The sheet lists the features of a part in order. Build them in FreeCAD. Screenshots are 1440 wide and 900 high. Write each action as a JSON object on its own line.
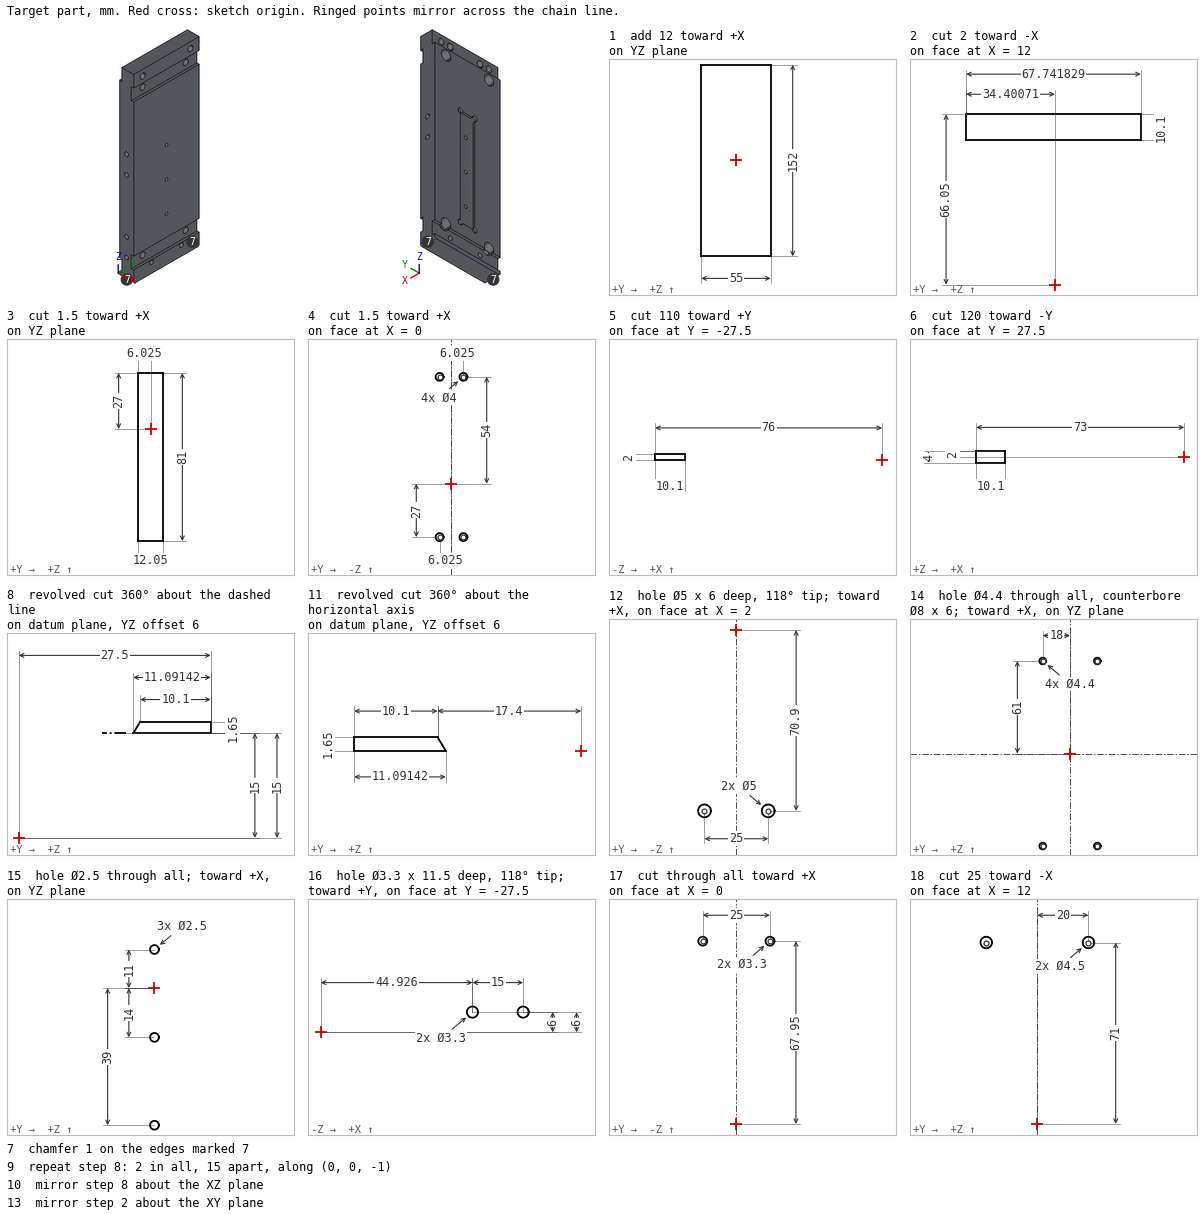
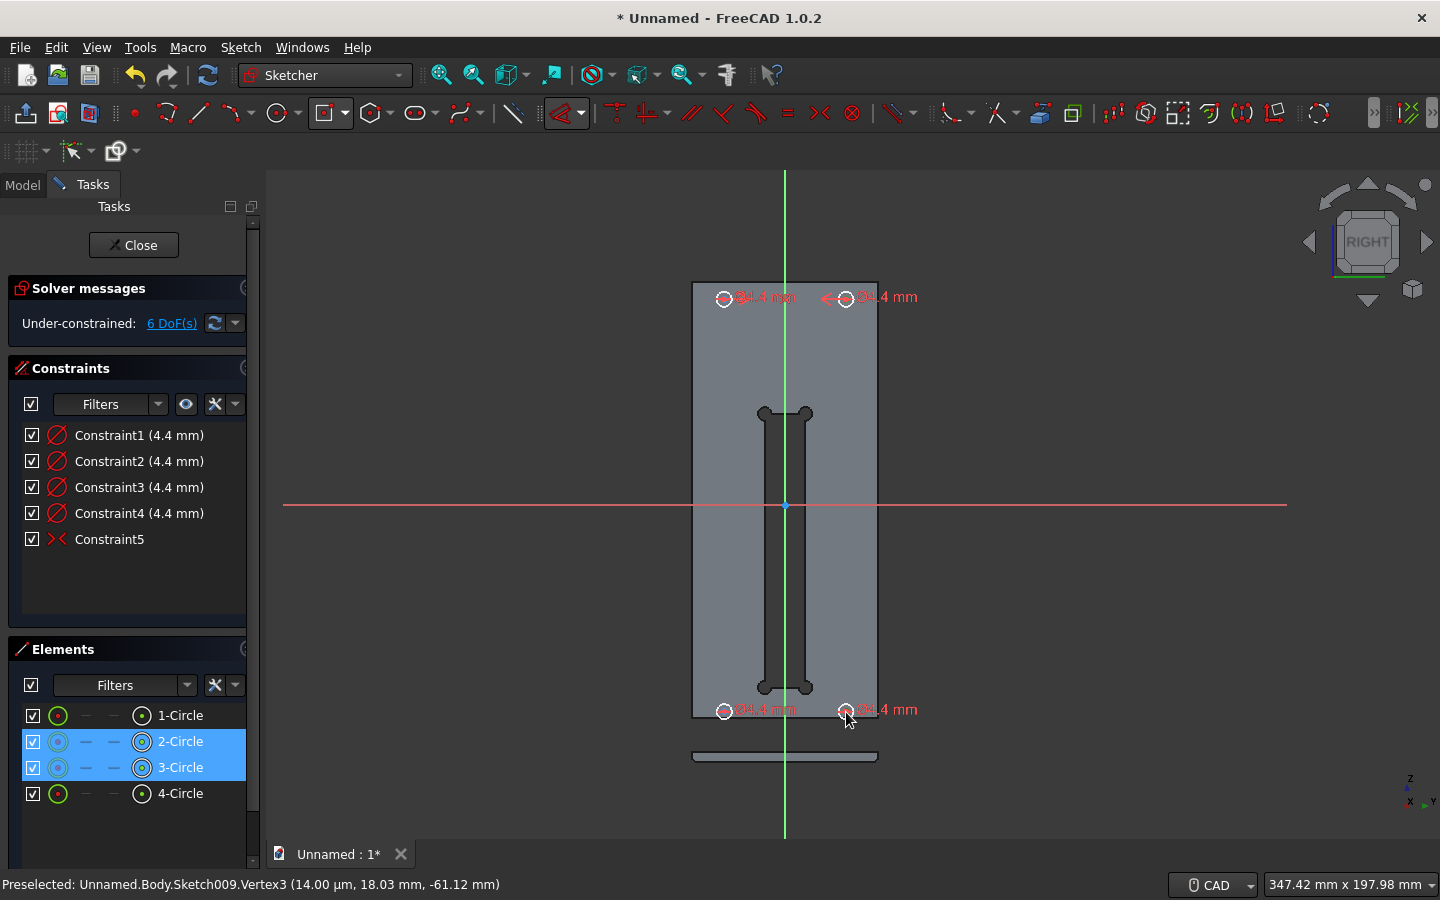
{"action": "left_click", "coordinate": [364, 505]}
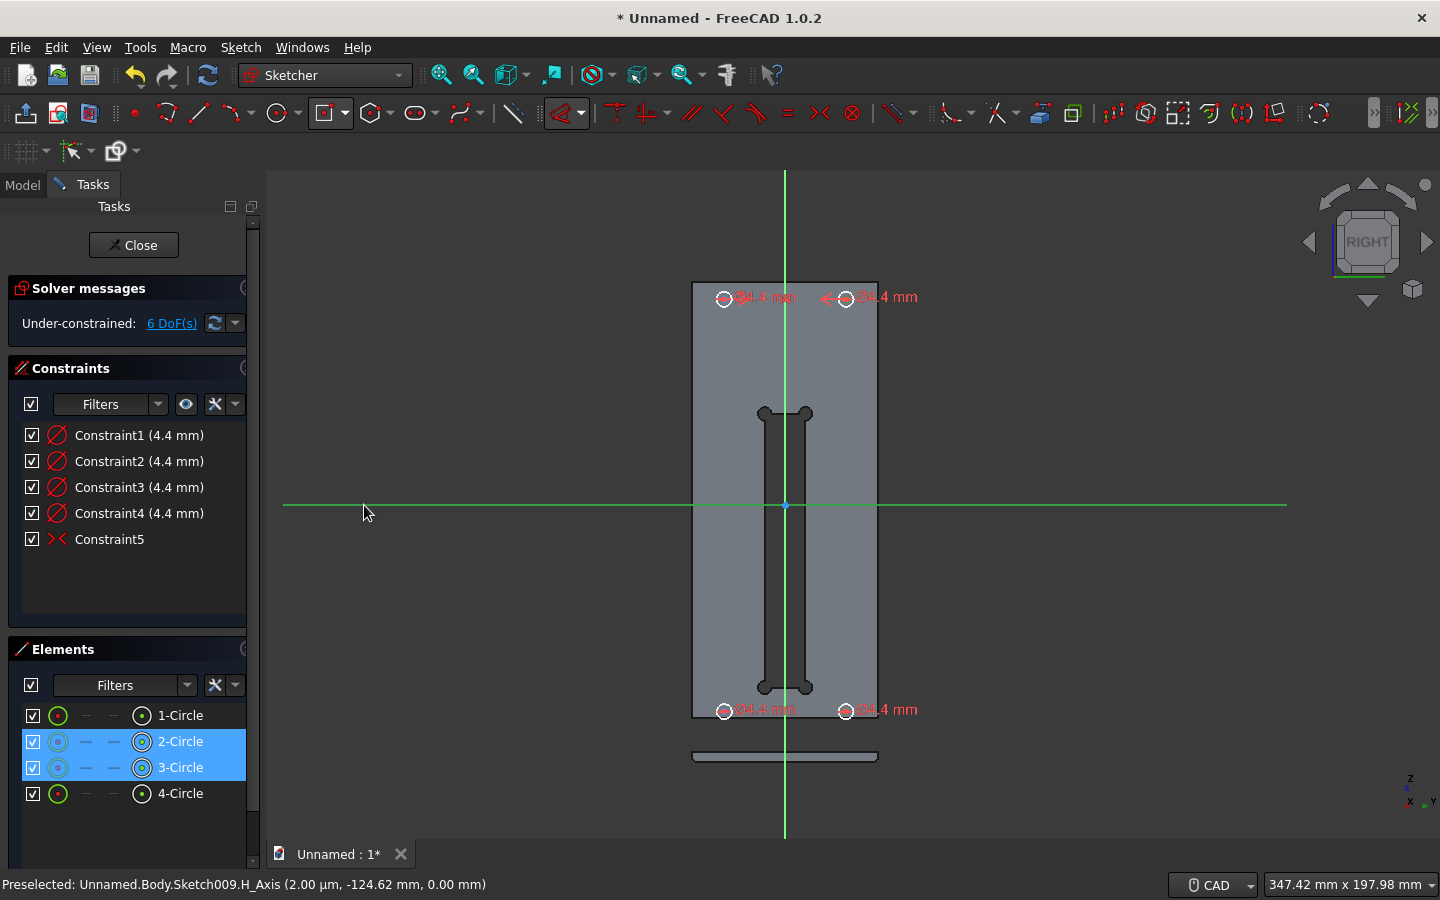
{"action": "left_click", "coordinate": [820, 114]}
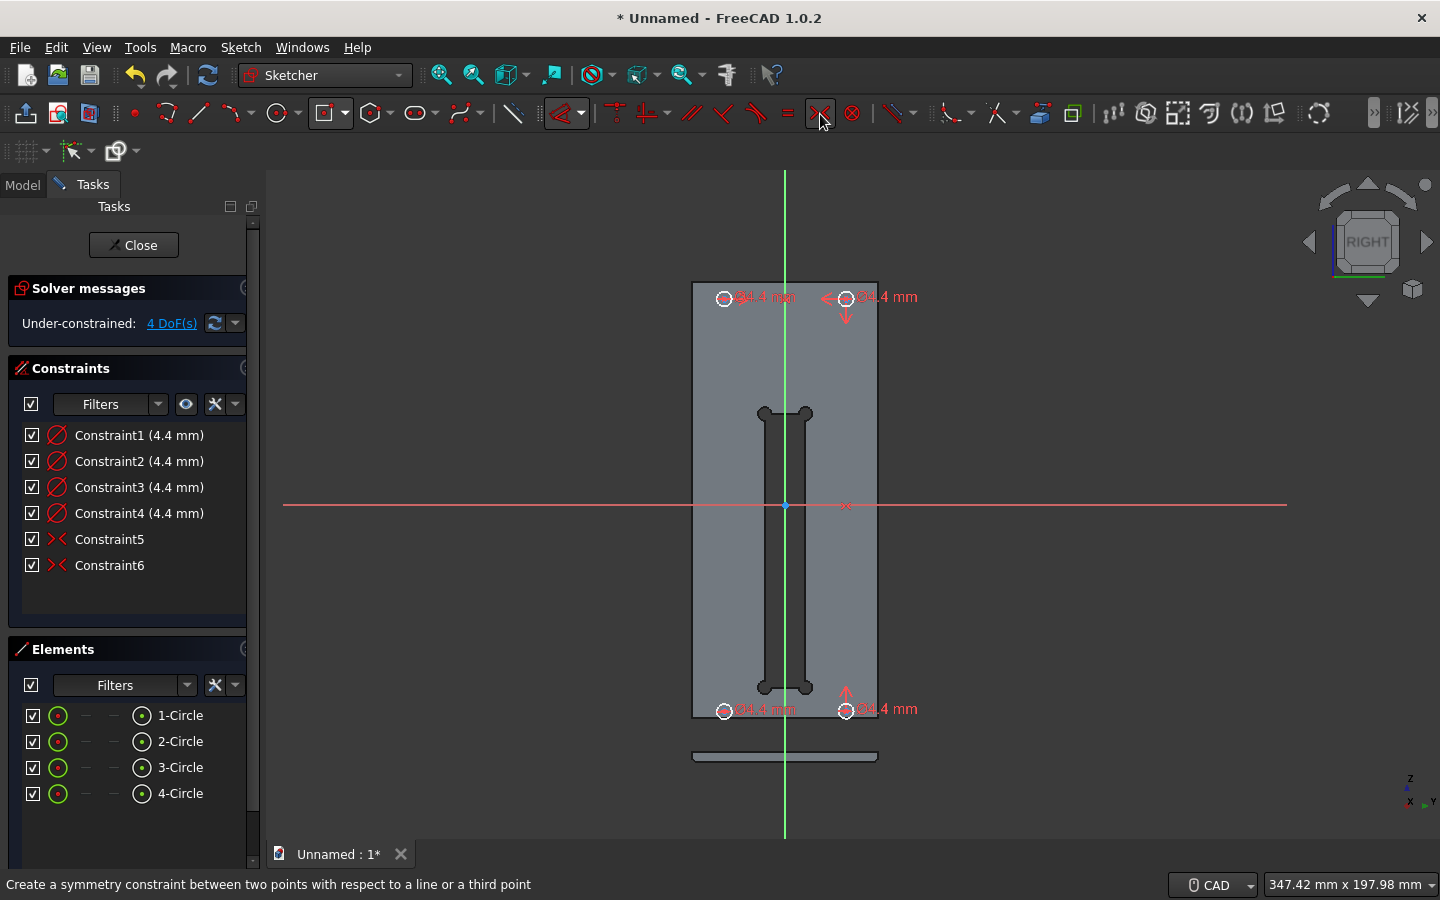
{"action": "left_click", "coordinate": [724, 299]}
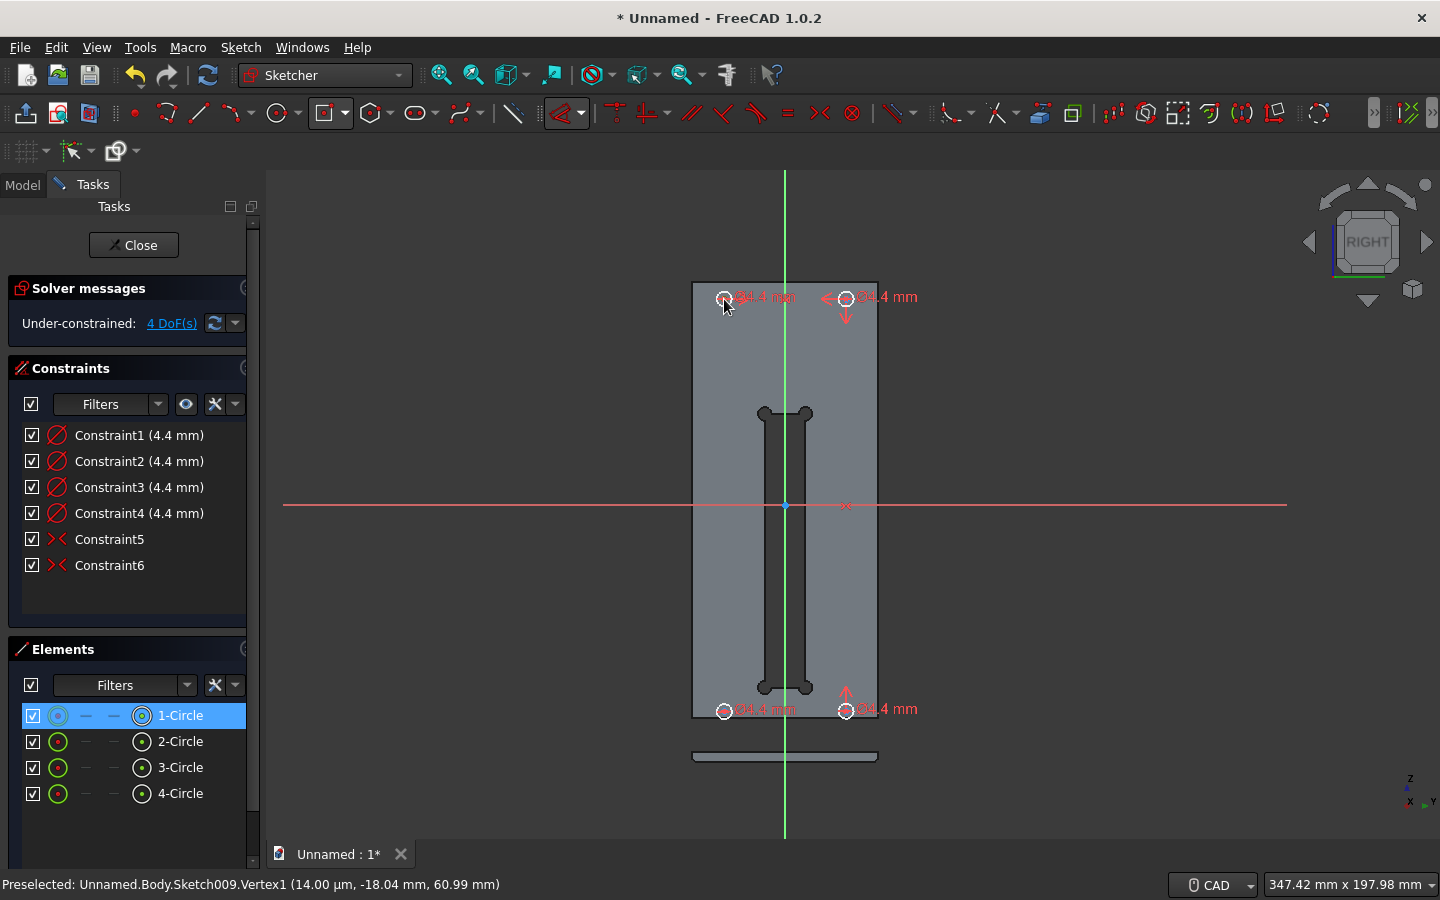
{"action": "left_click", "coordinate": [724, 712]}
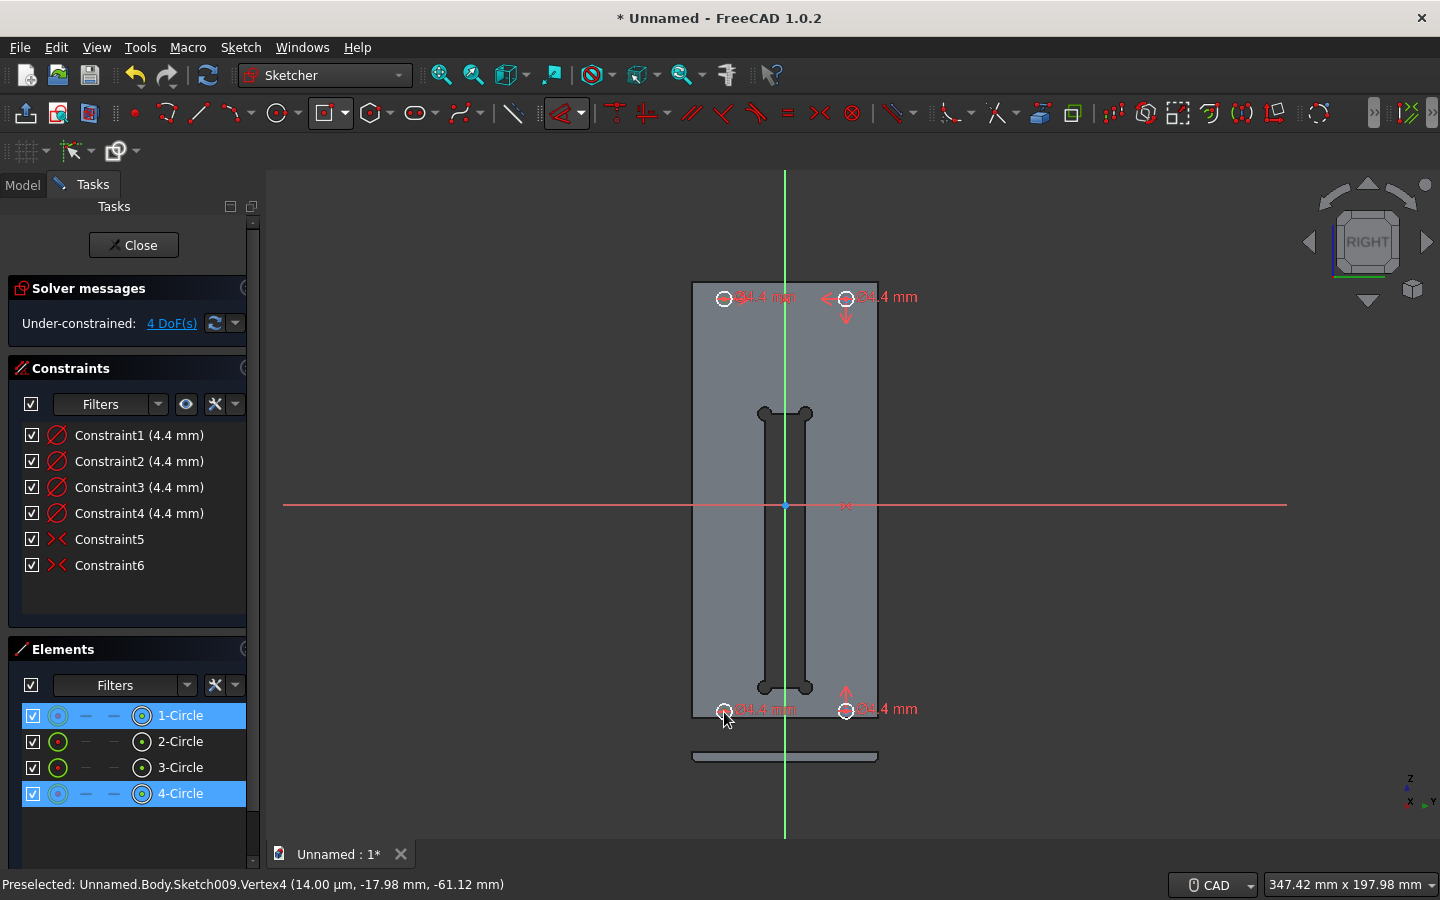
{"action": "left_click", "coordinate": [364, 505]}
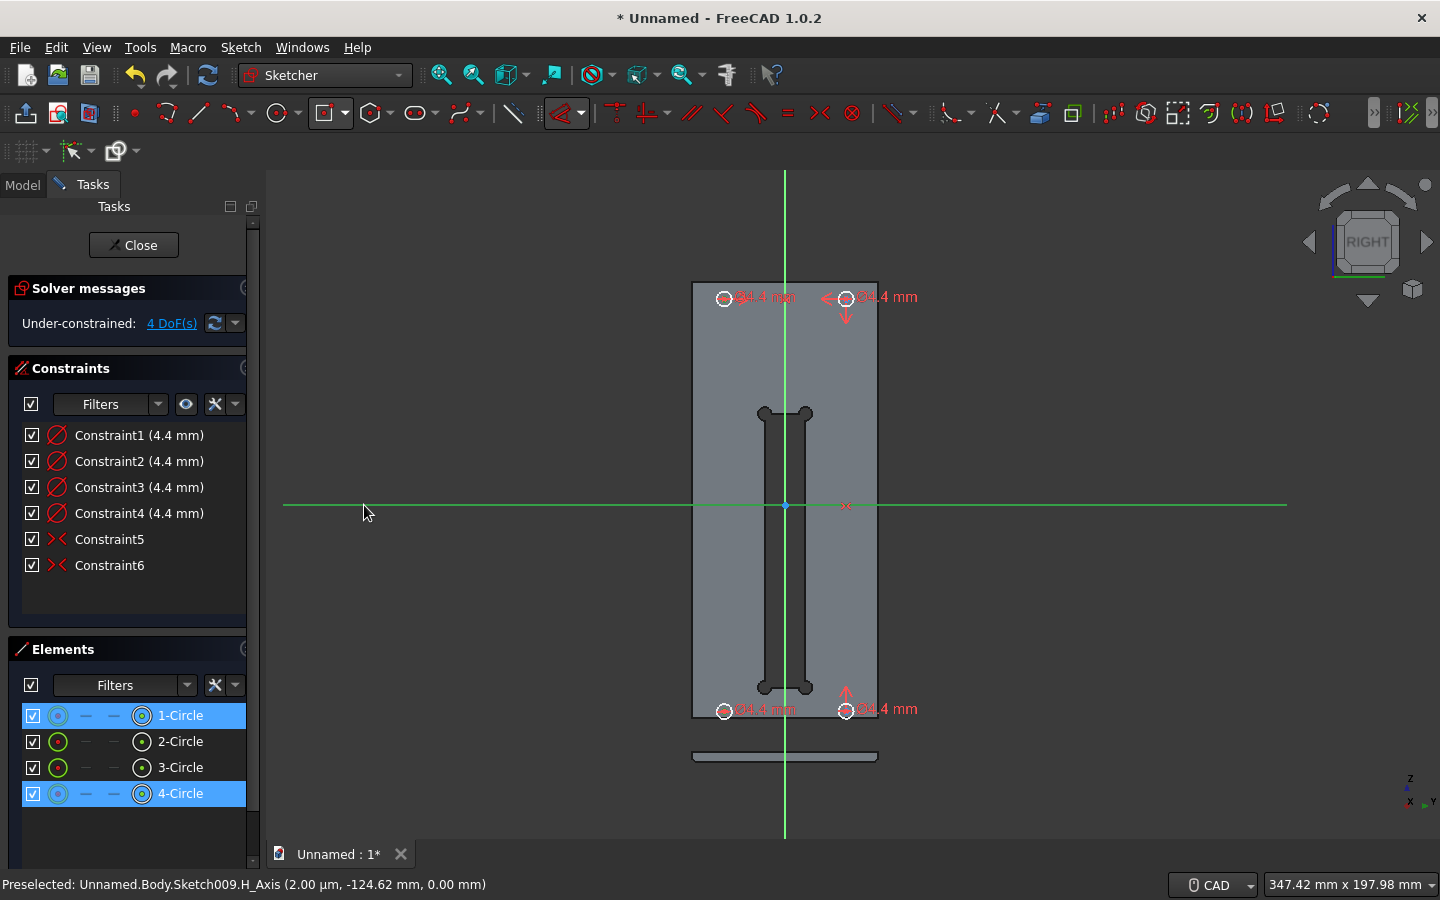
{"action": "left_click", "coordinate": [820, 114]}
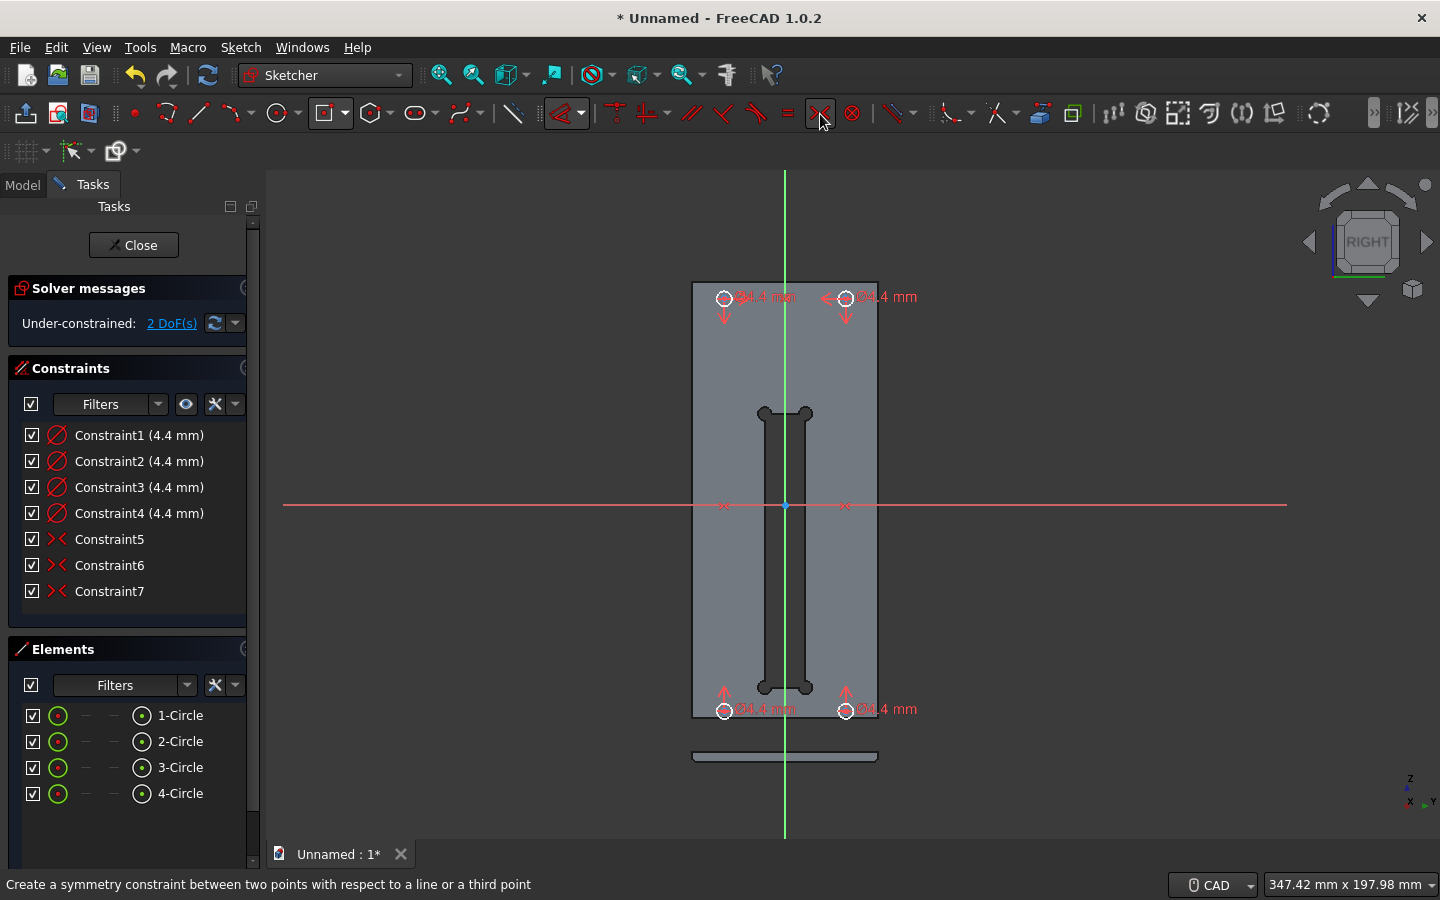
{"action": "left_click", "coordinate": [724, 299]}